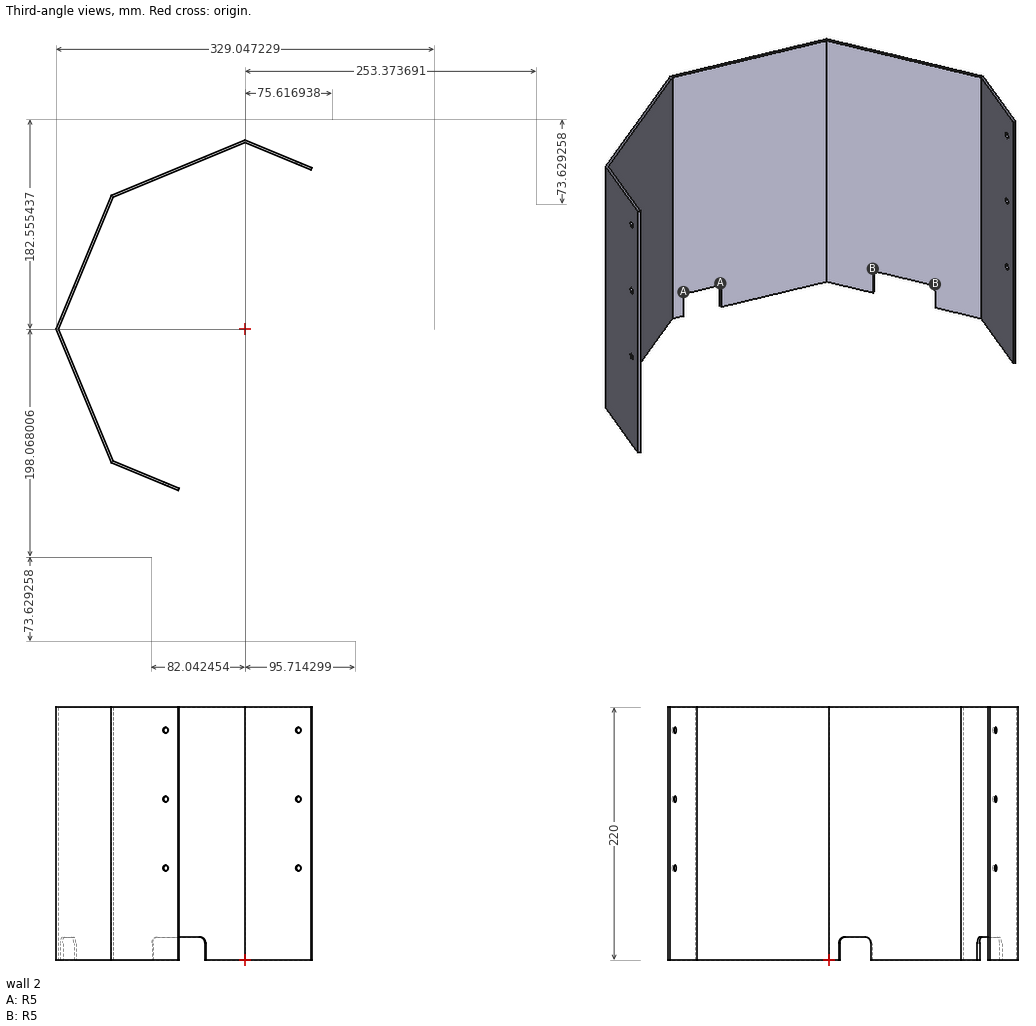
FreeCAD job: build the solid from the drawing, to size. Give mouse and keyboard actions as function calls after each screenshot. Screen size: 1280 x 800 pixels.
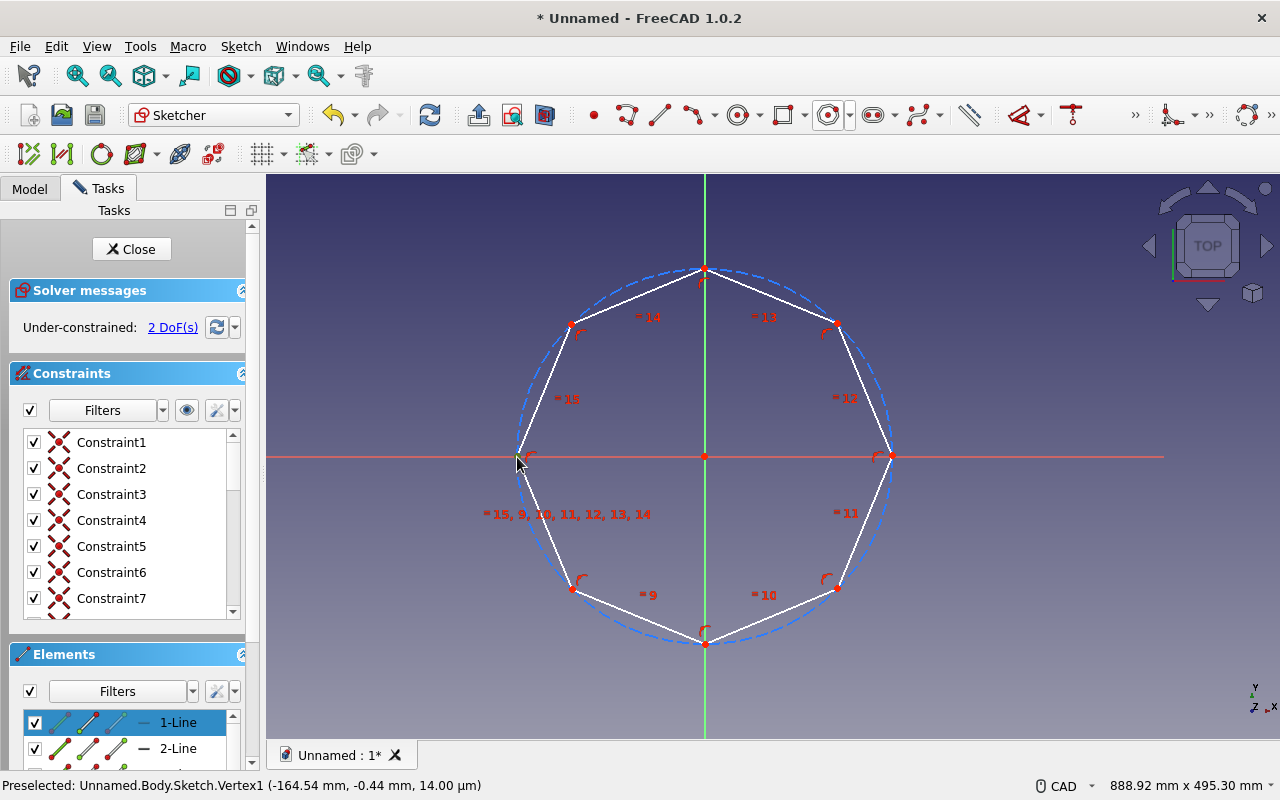
click(353, 456)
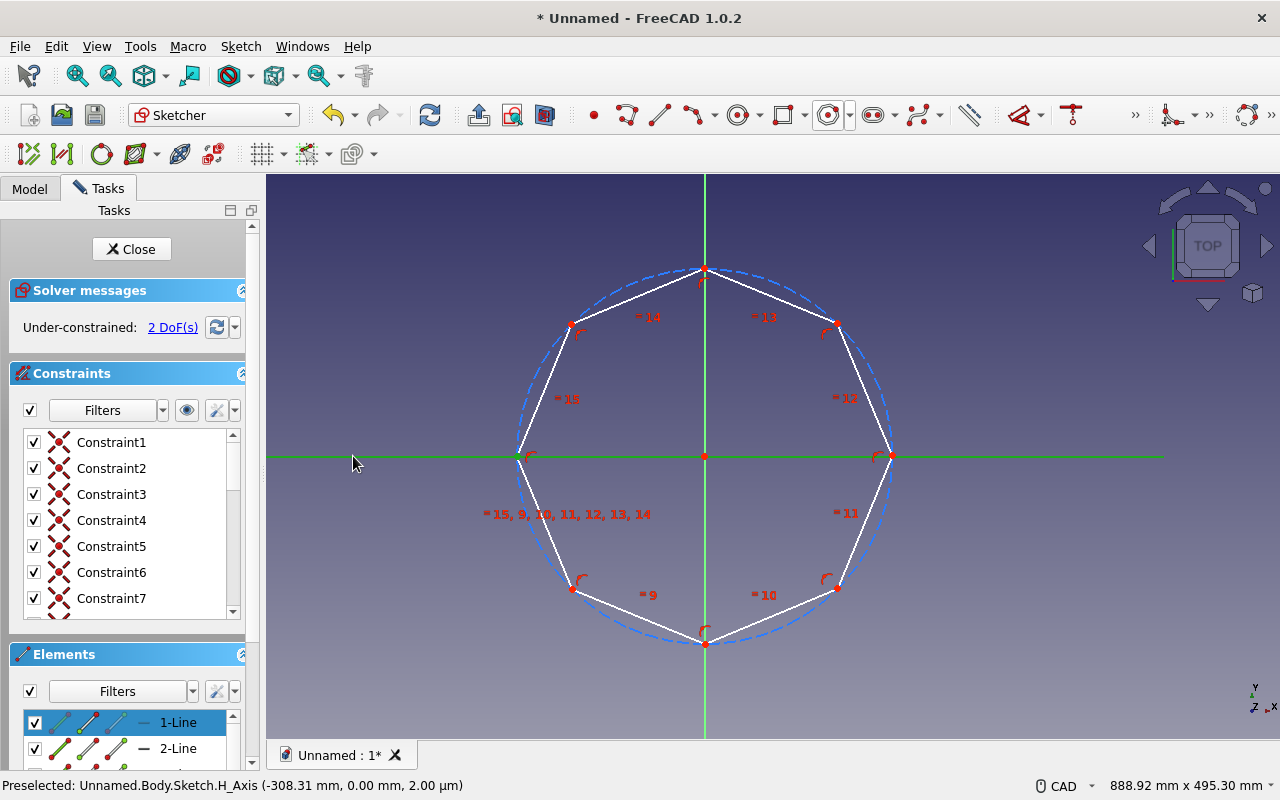
click(1071, 116)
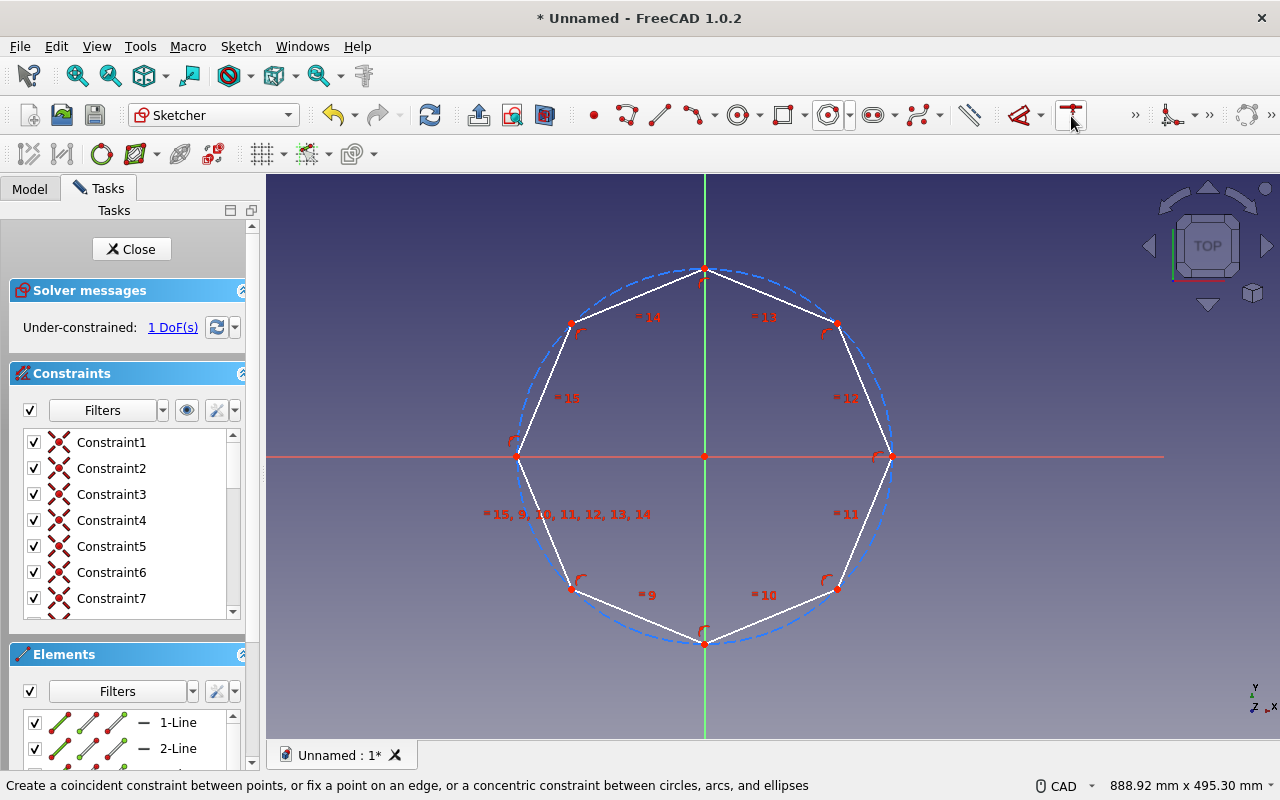
click(517, 456)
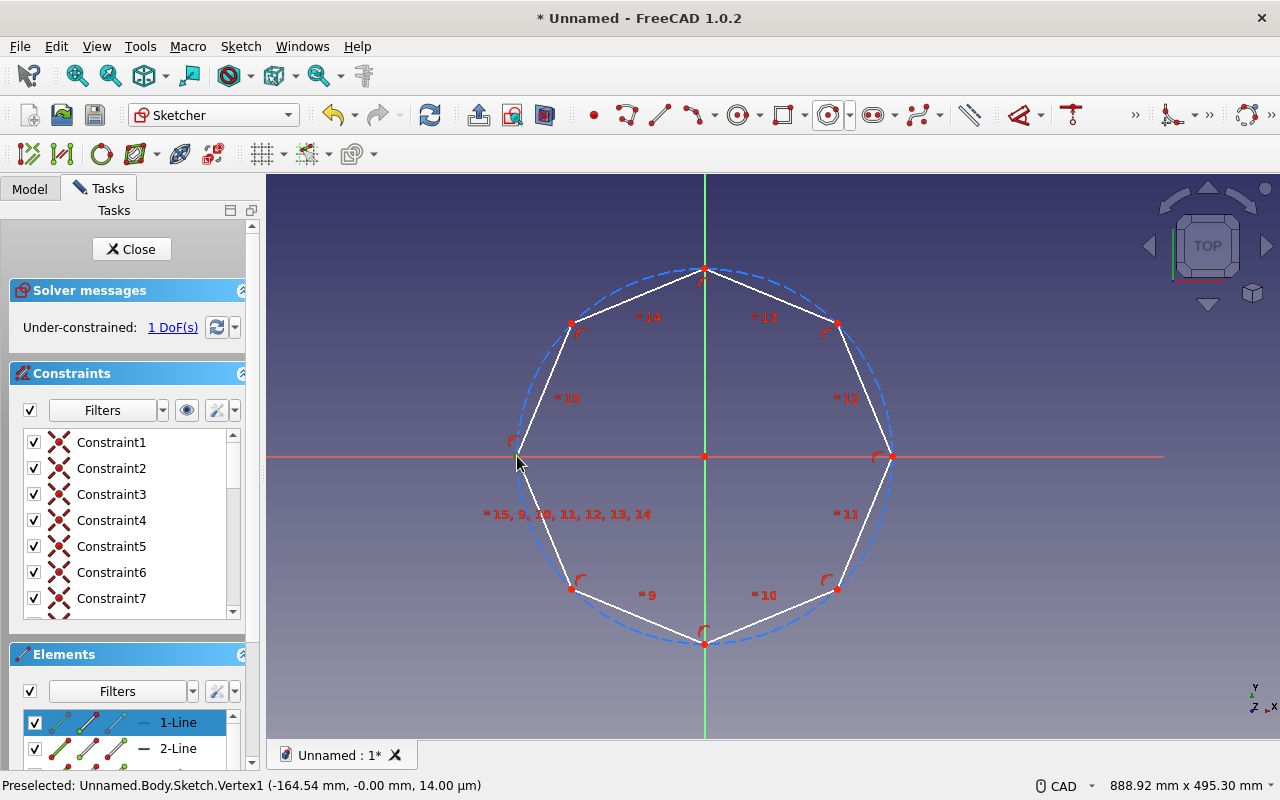
click(892, 456)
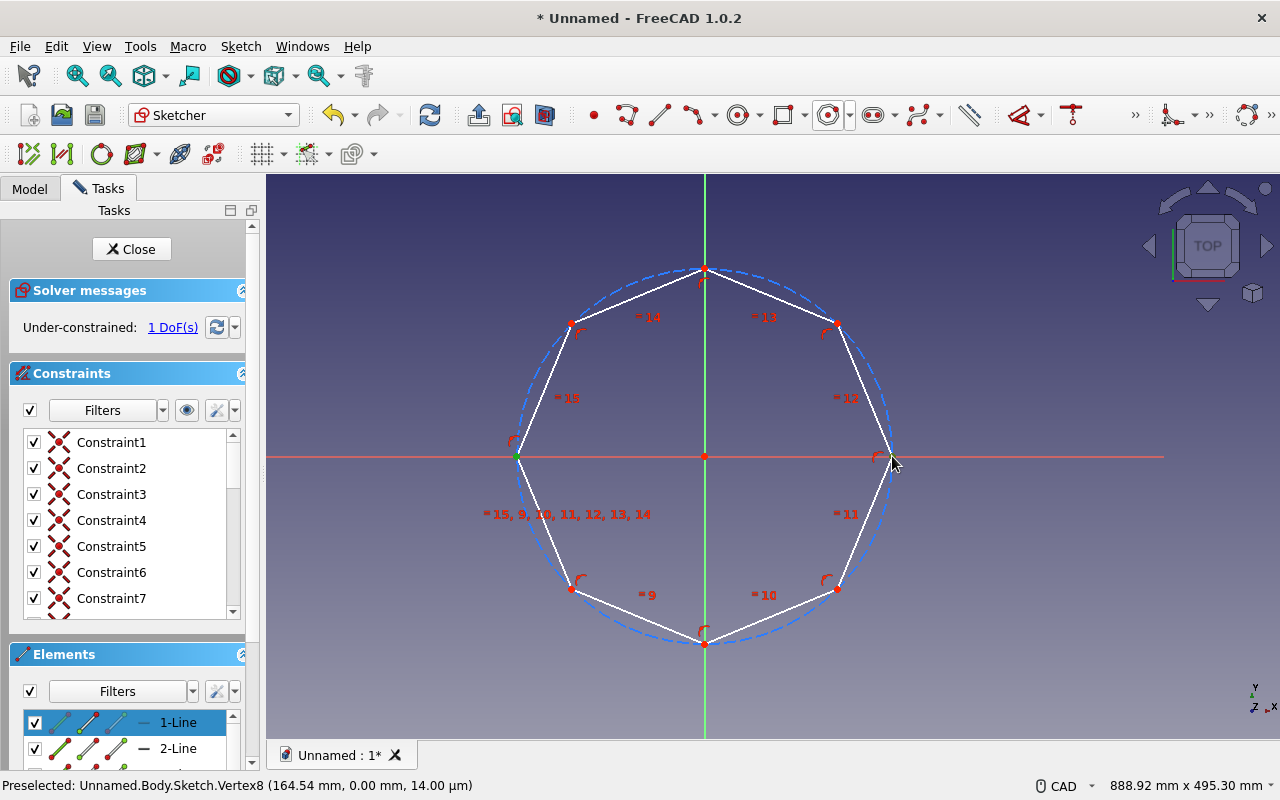
click(1040, 116)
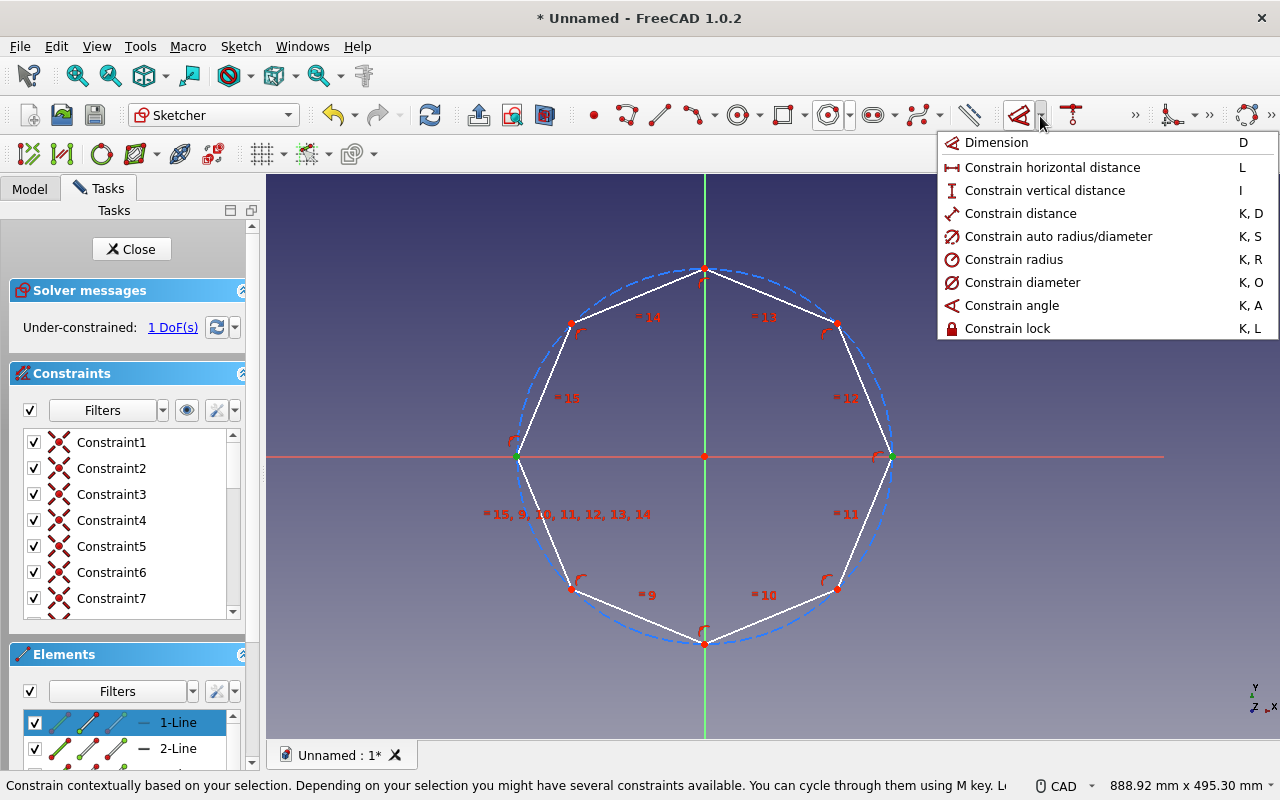
click(1108, 168)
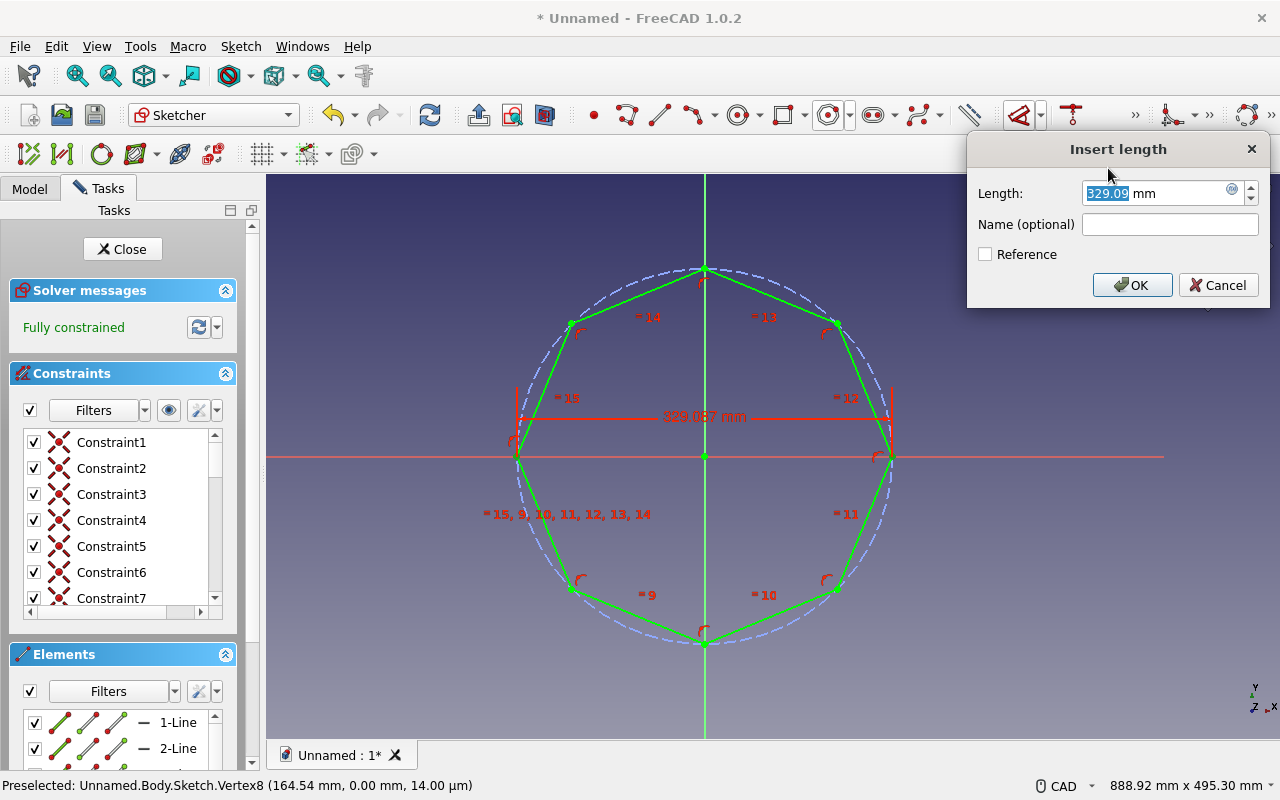
text(329.047229)
key(Return)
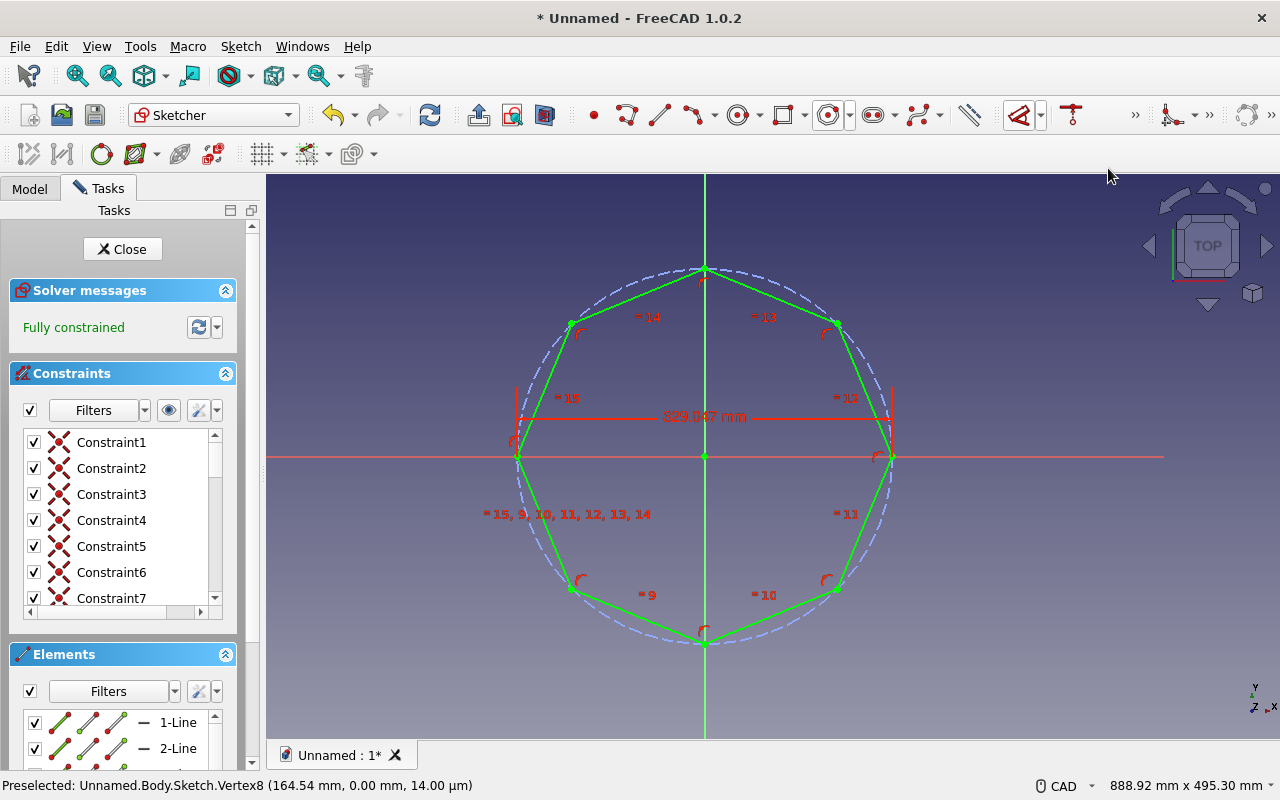
click(123, 249)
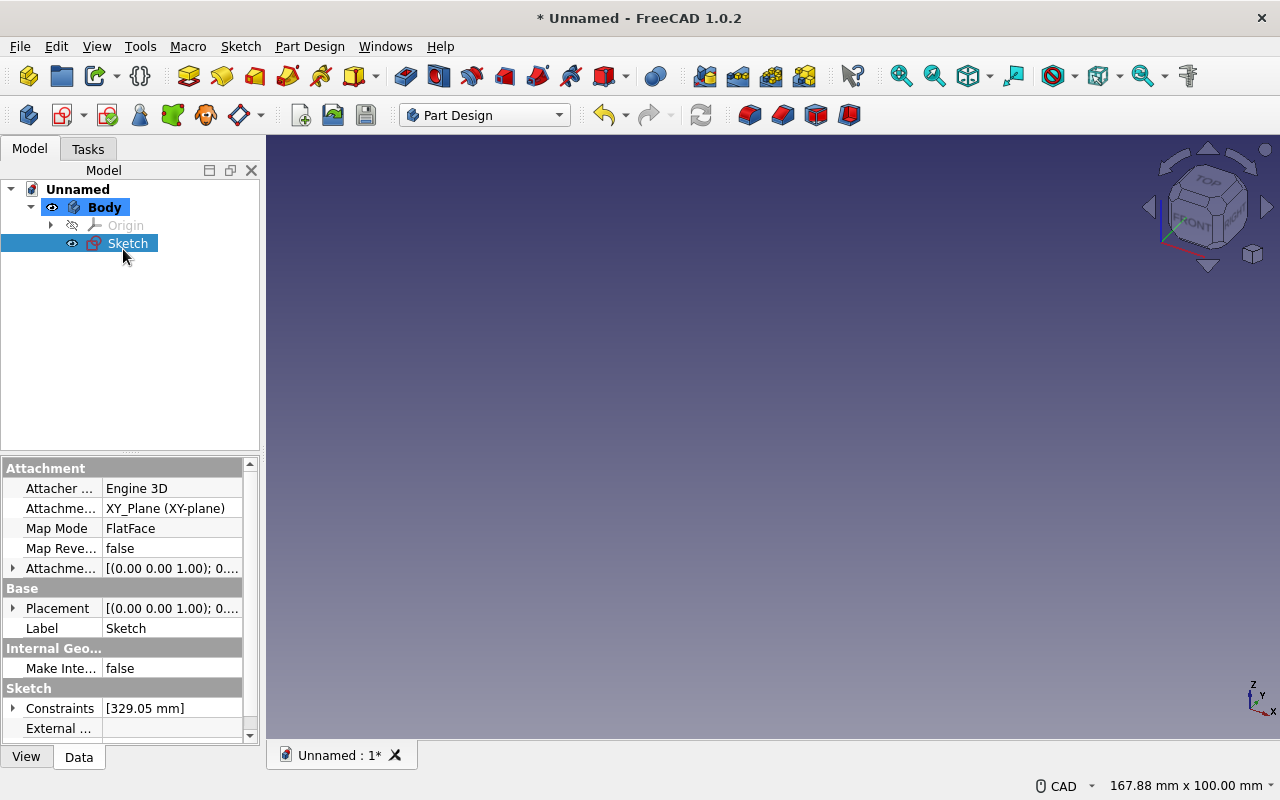
click(189, 76)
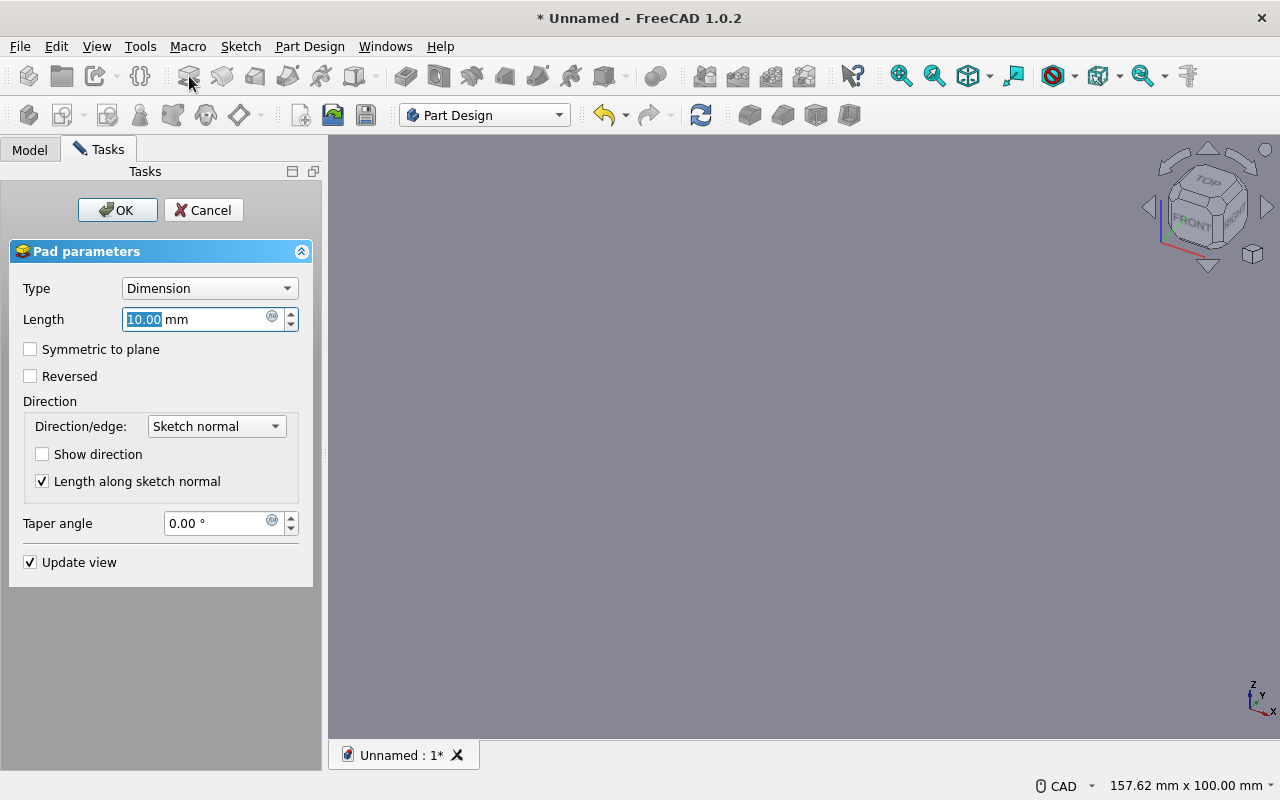
text(220)
key(Tab)